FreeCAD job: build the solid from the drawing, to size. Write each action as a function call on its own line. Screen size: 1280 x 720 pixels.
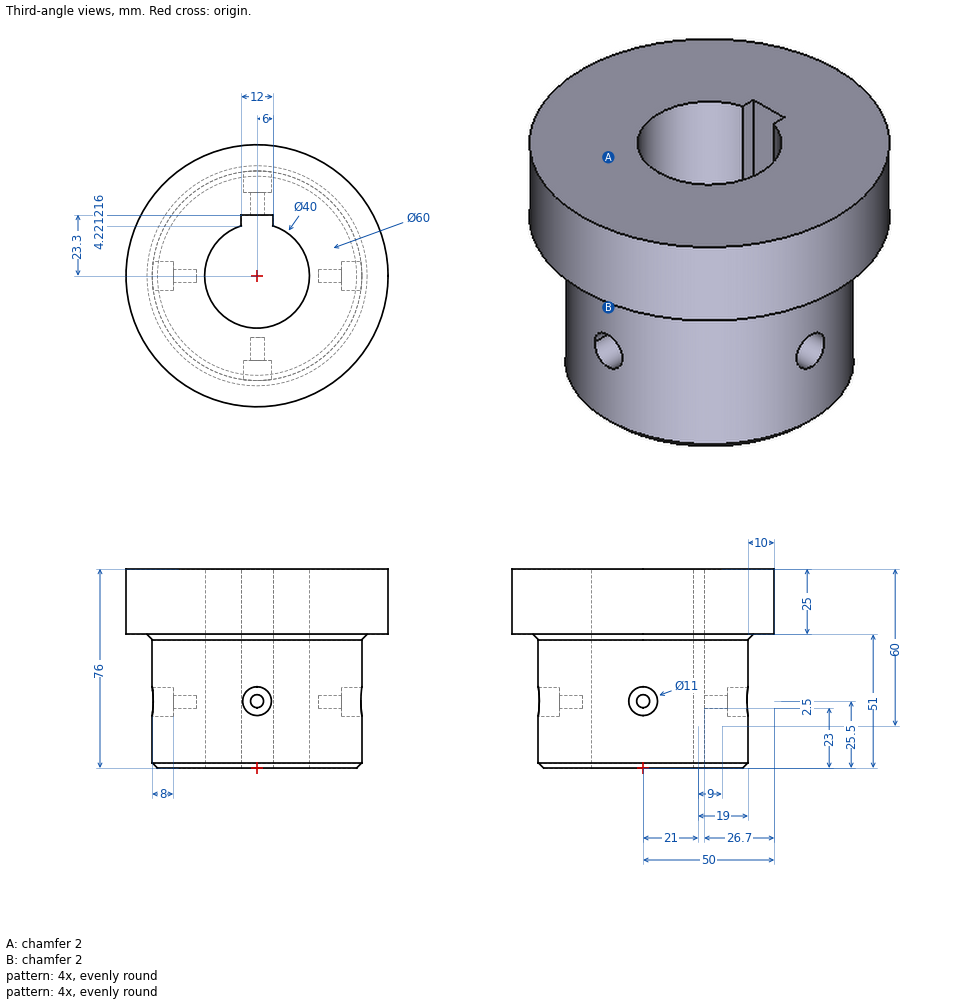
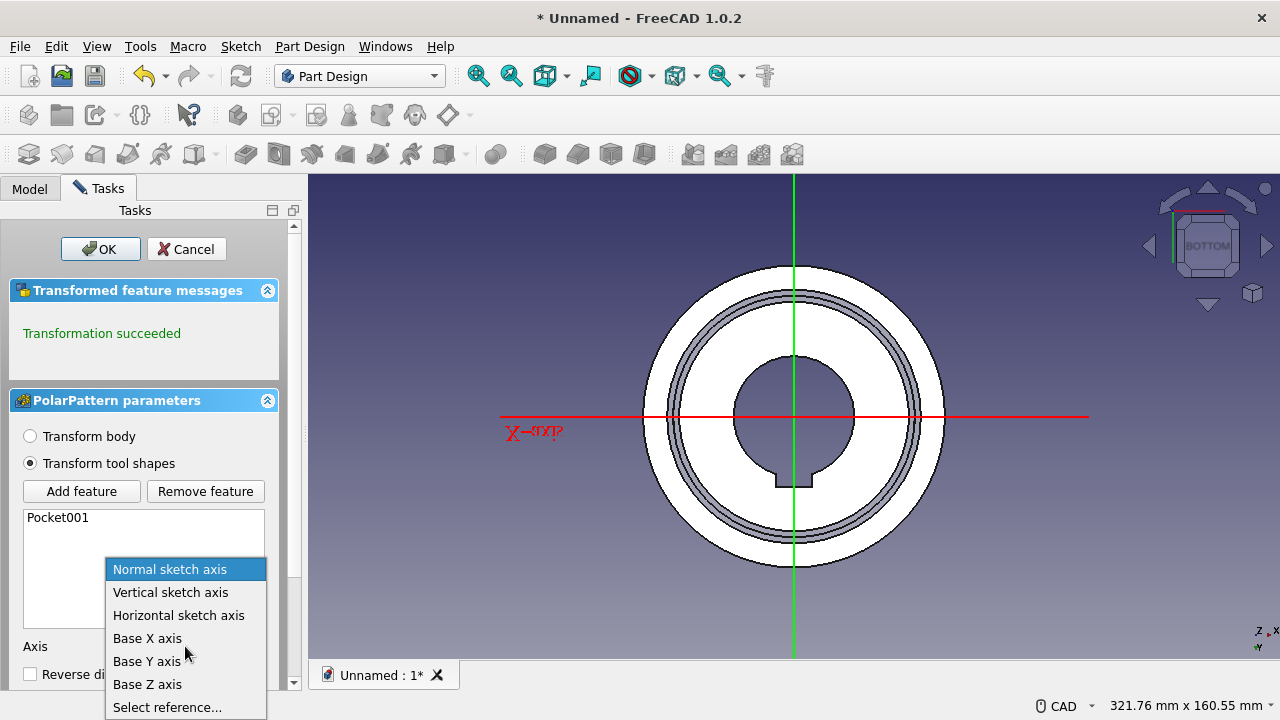
click(184, 684)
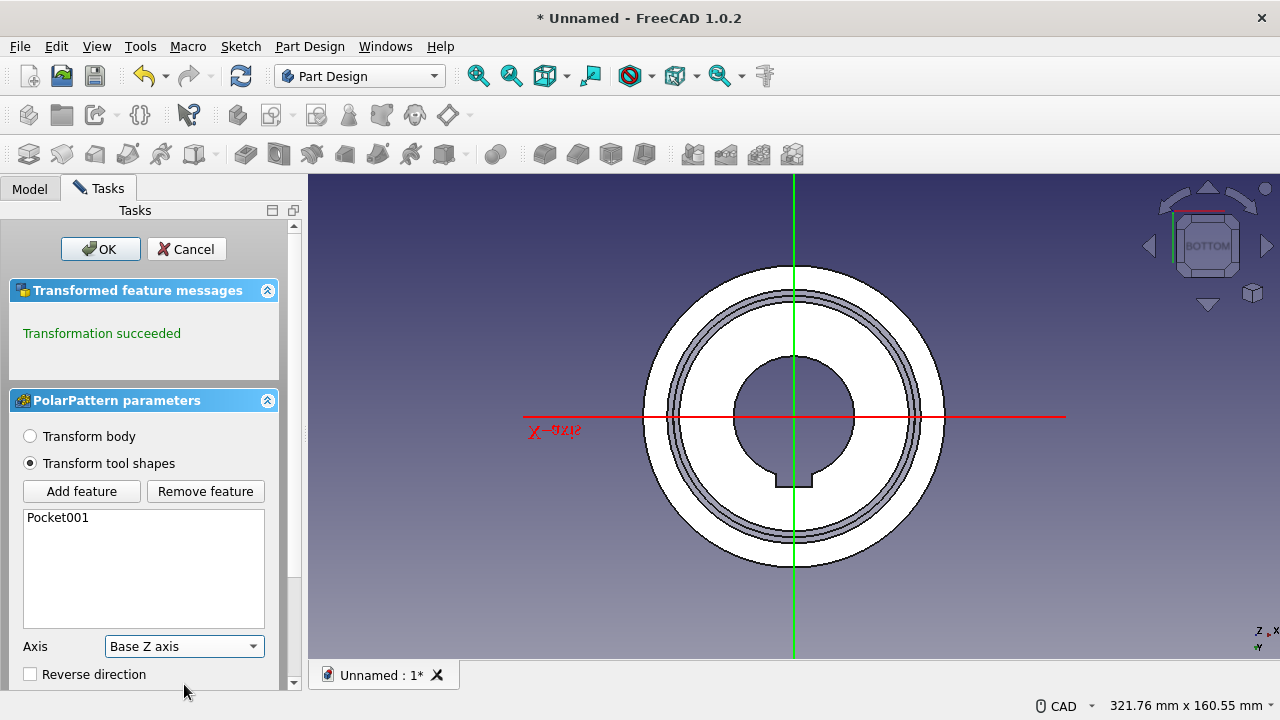
scroll(294, 455, down, 3)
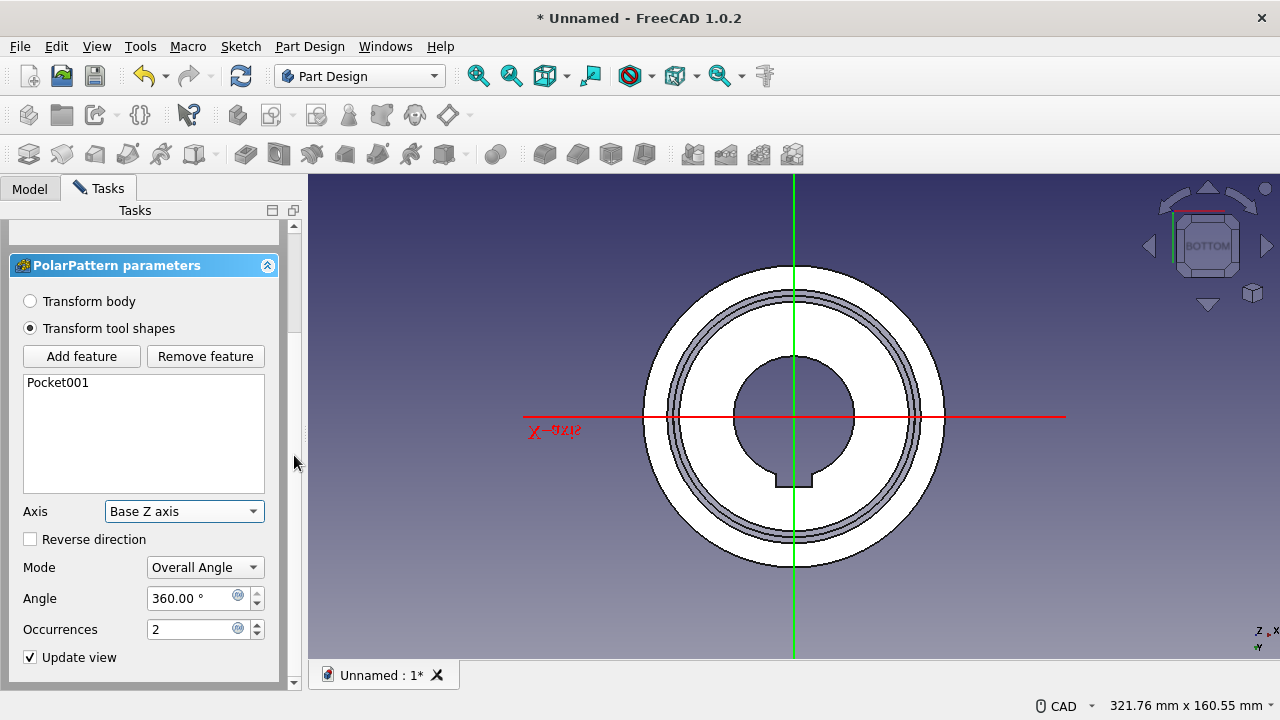
triple_click(199, 630)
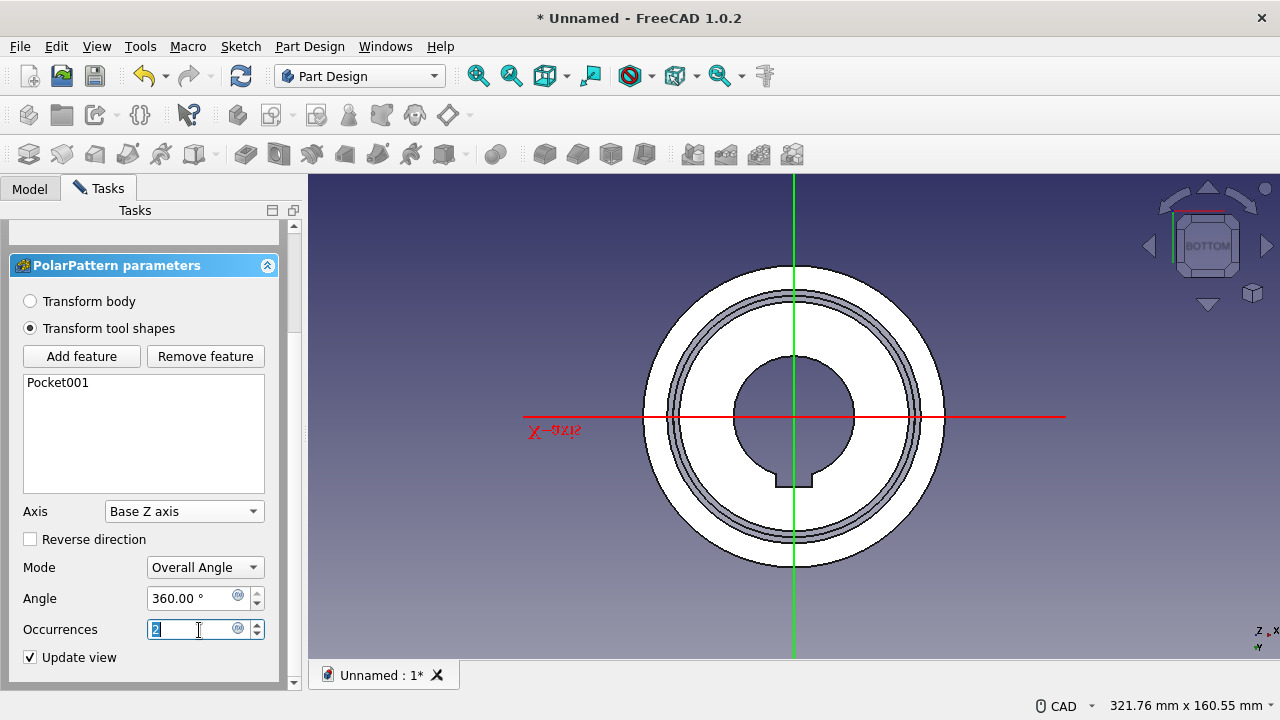
text(4)
key(Tab)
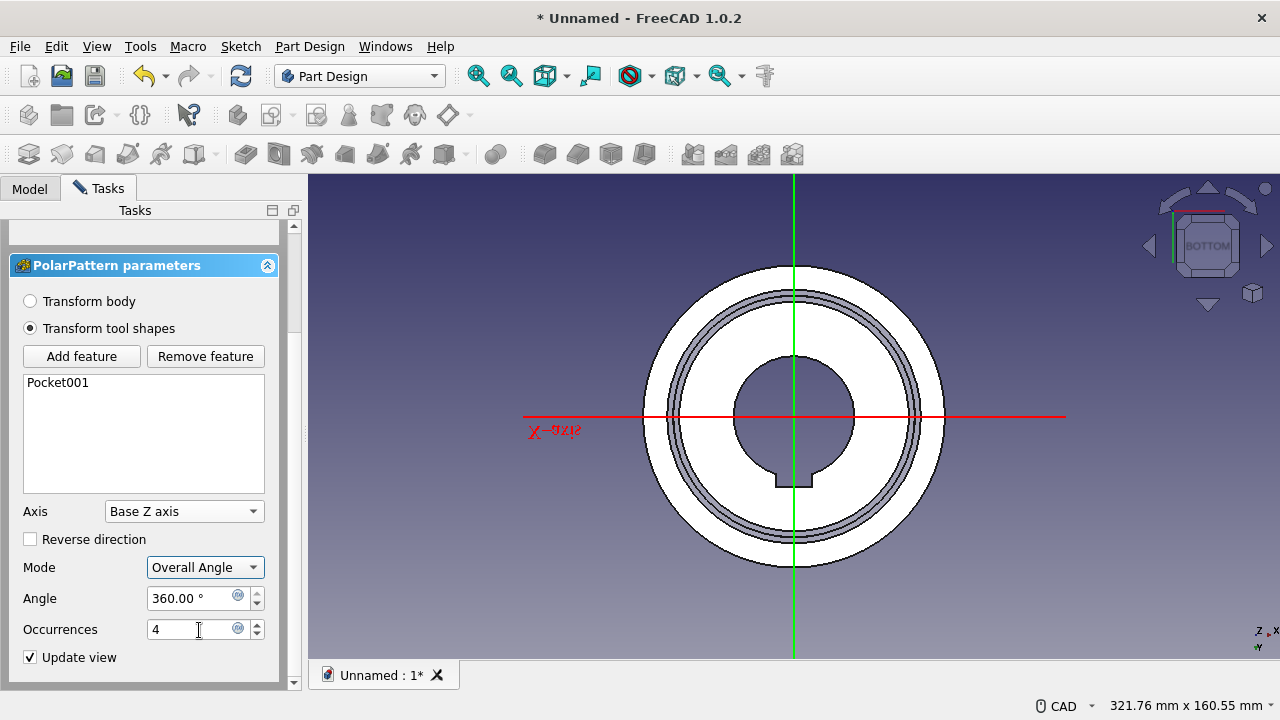
scroll(294, 455, up, 3)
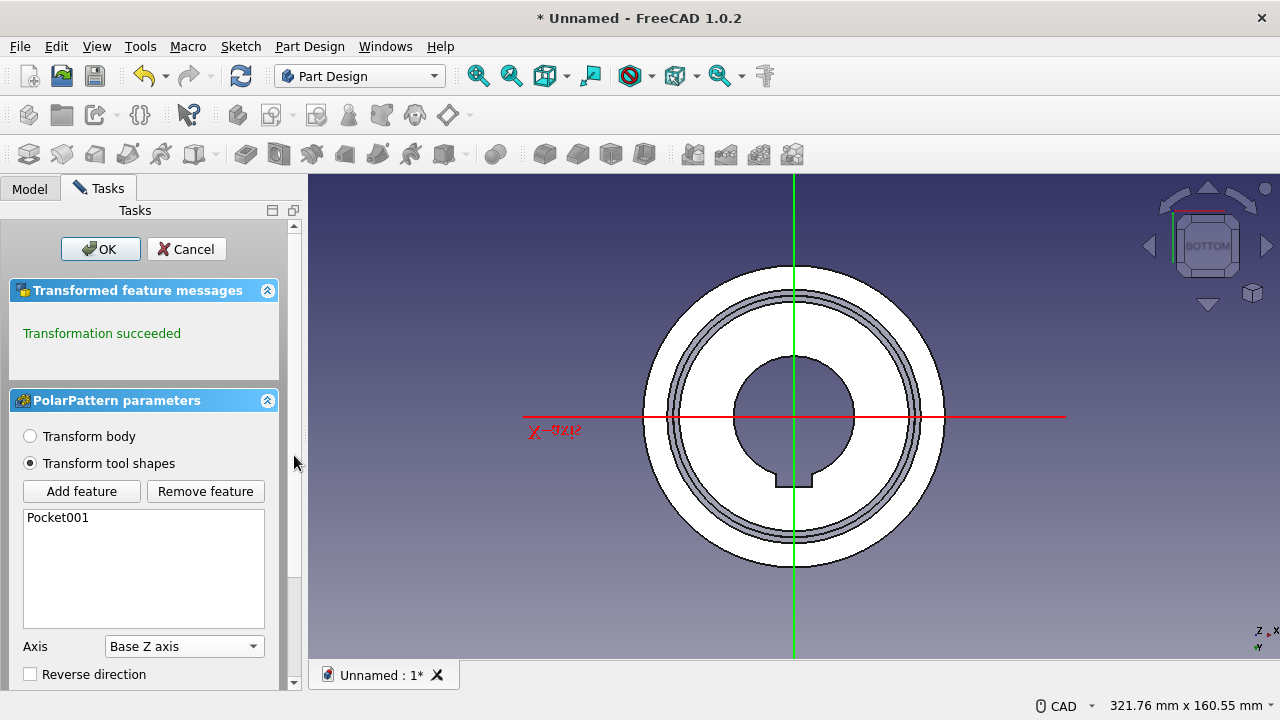
click(101, 249)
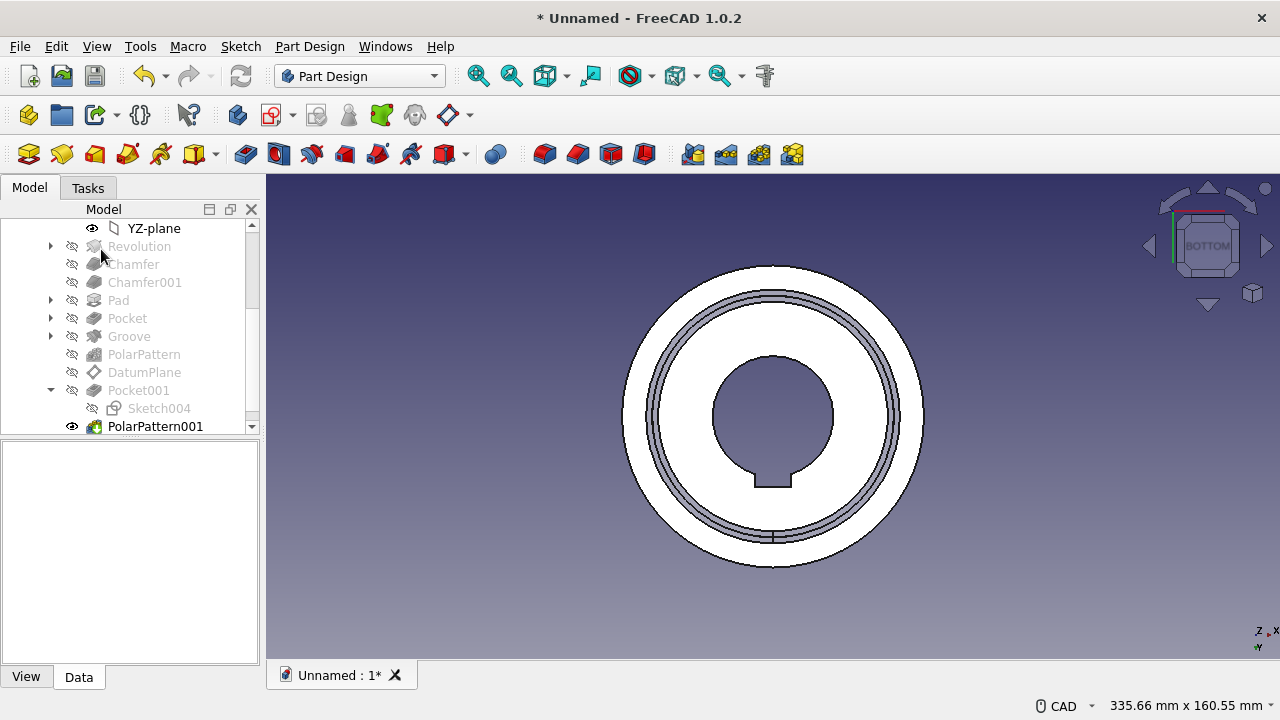
key(0)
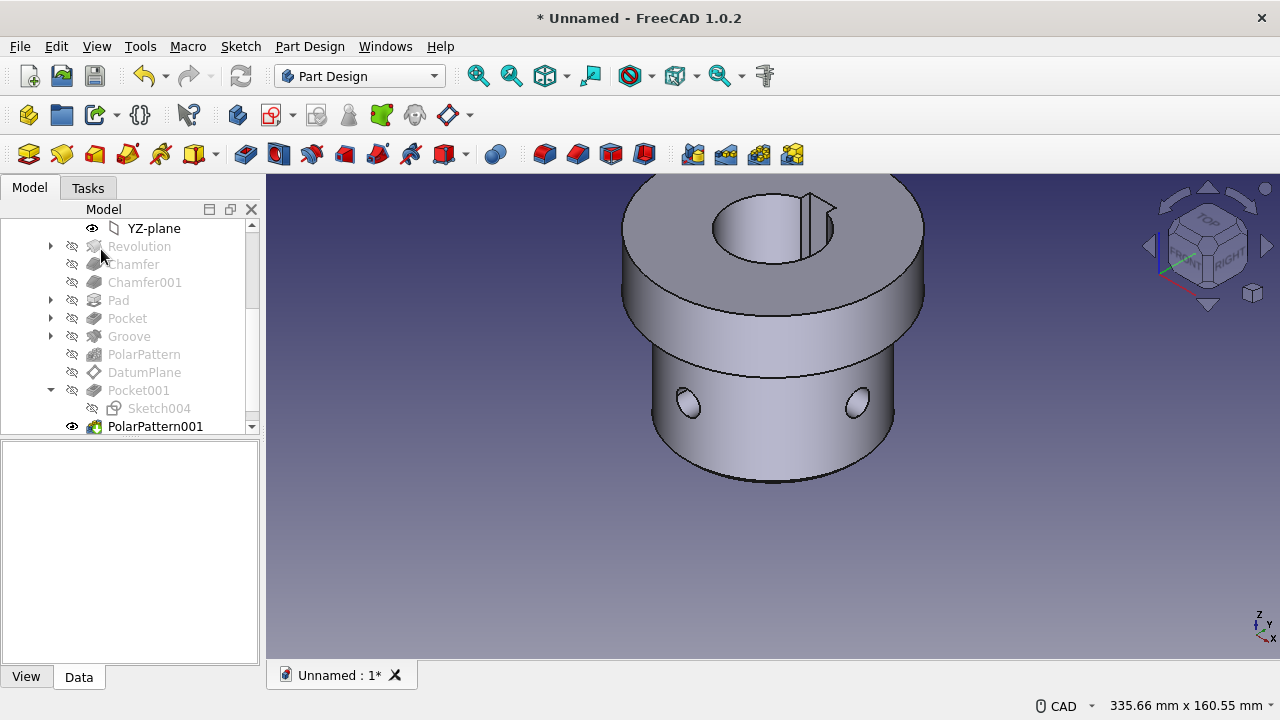
key(v)
key(f)